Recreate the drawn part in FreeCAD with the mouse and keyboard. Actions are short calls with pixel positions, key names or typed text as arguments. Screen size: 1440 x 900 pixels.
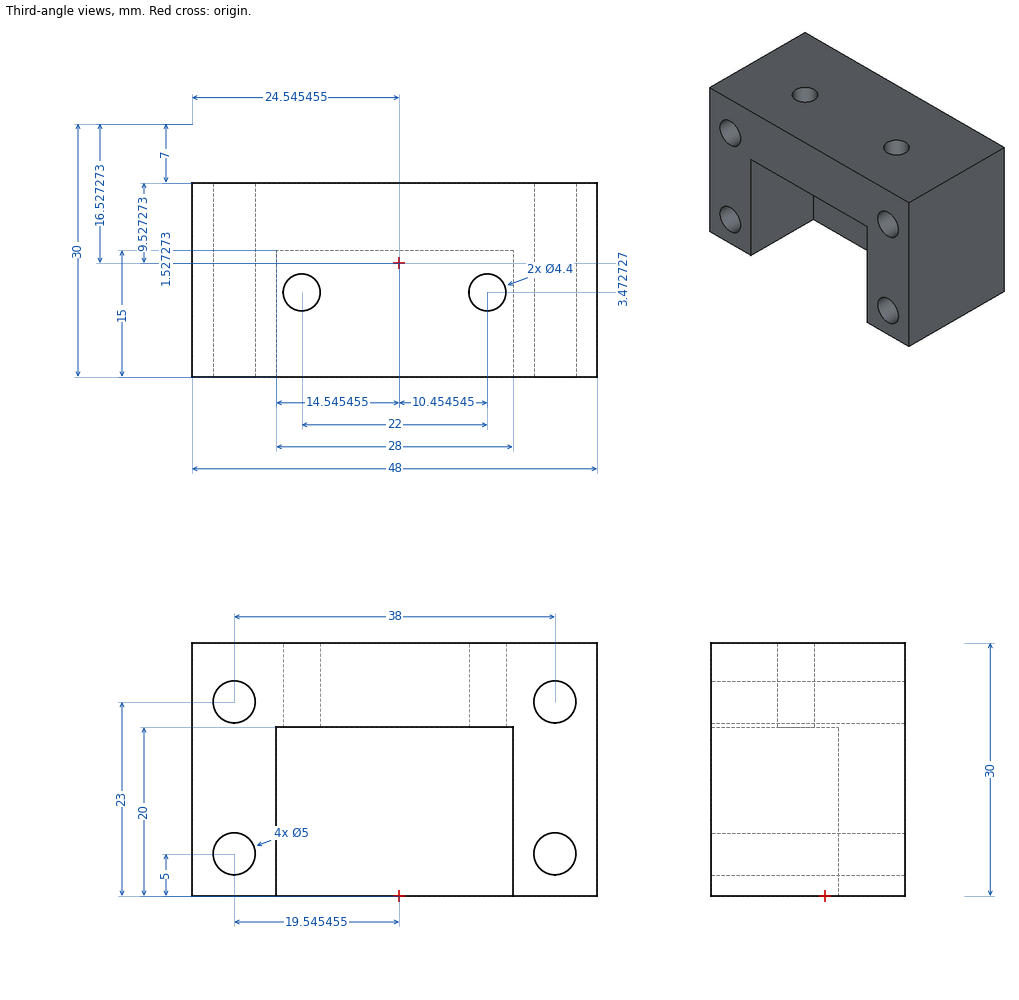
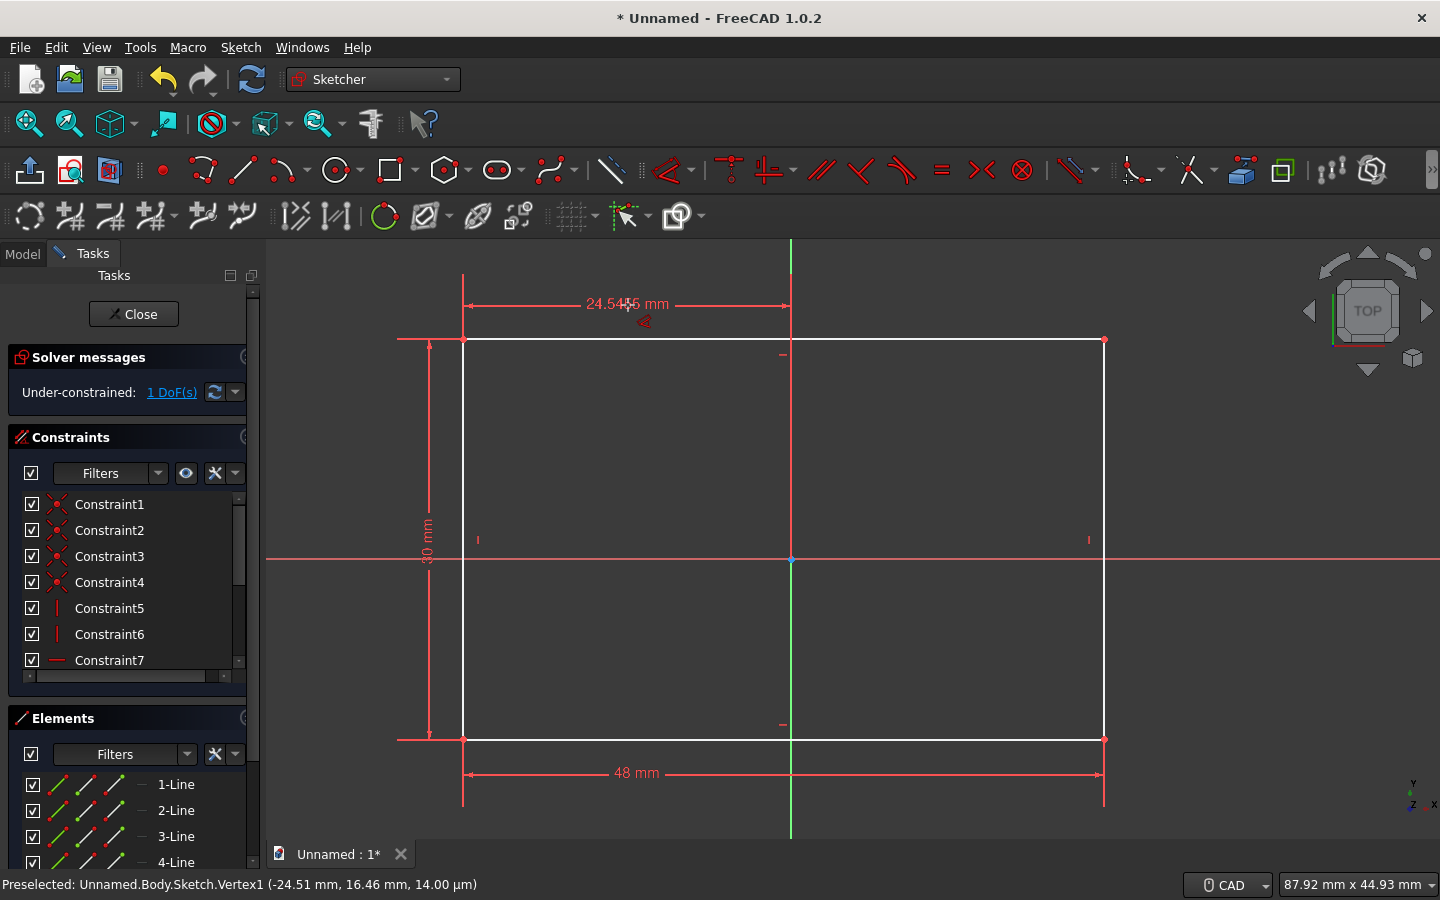
click(464, 339)
click(430, 449)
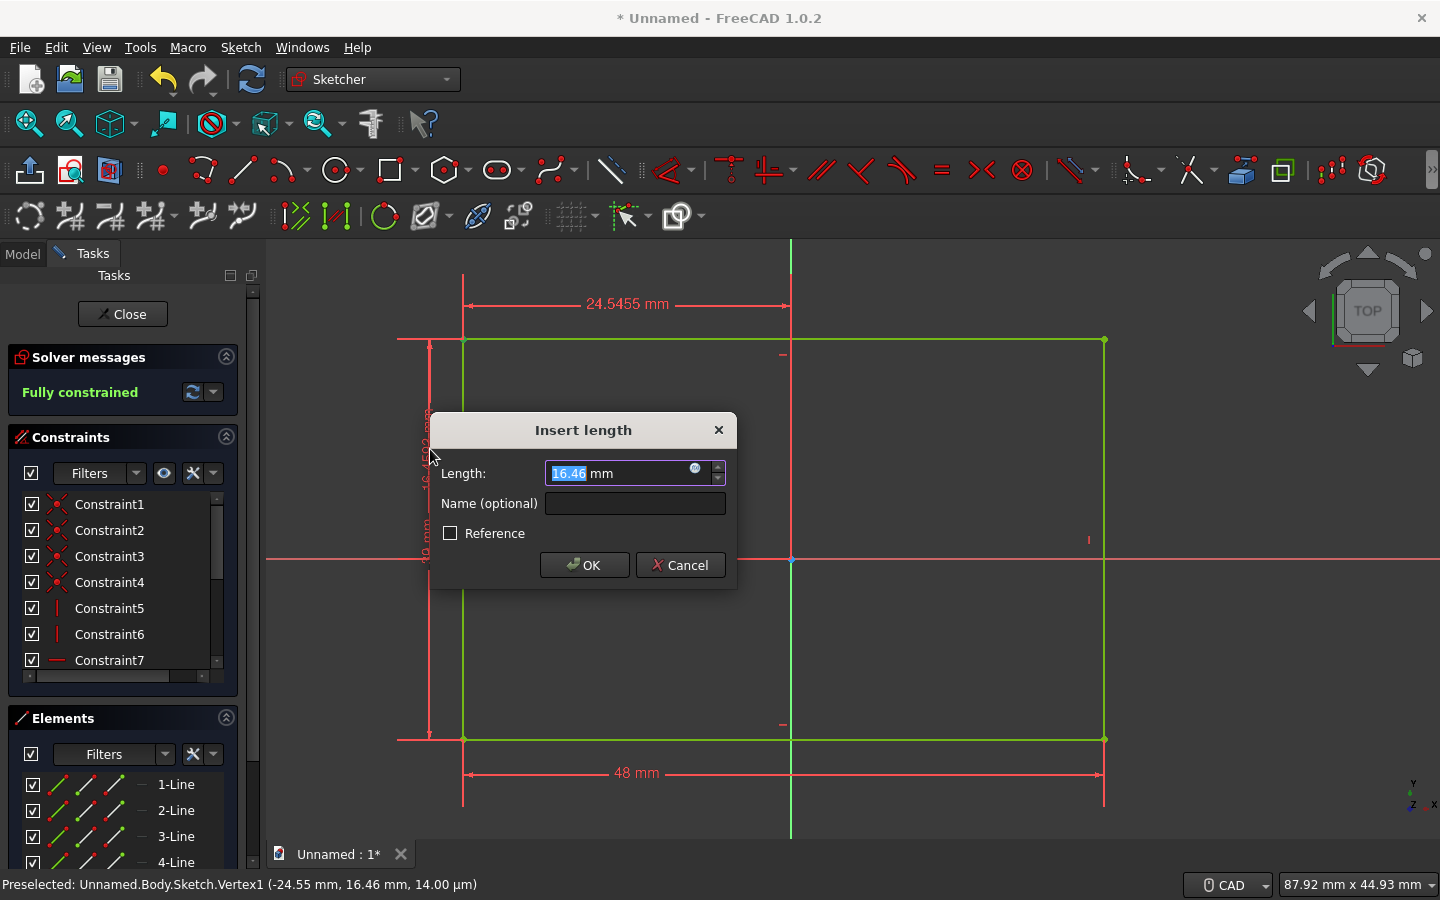
text(16.527273)
key(Return)
key(Escape)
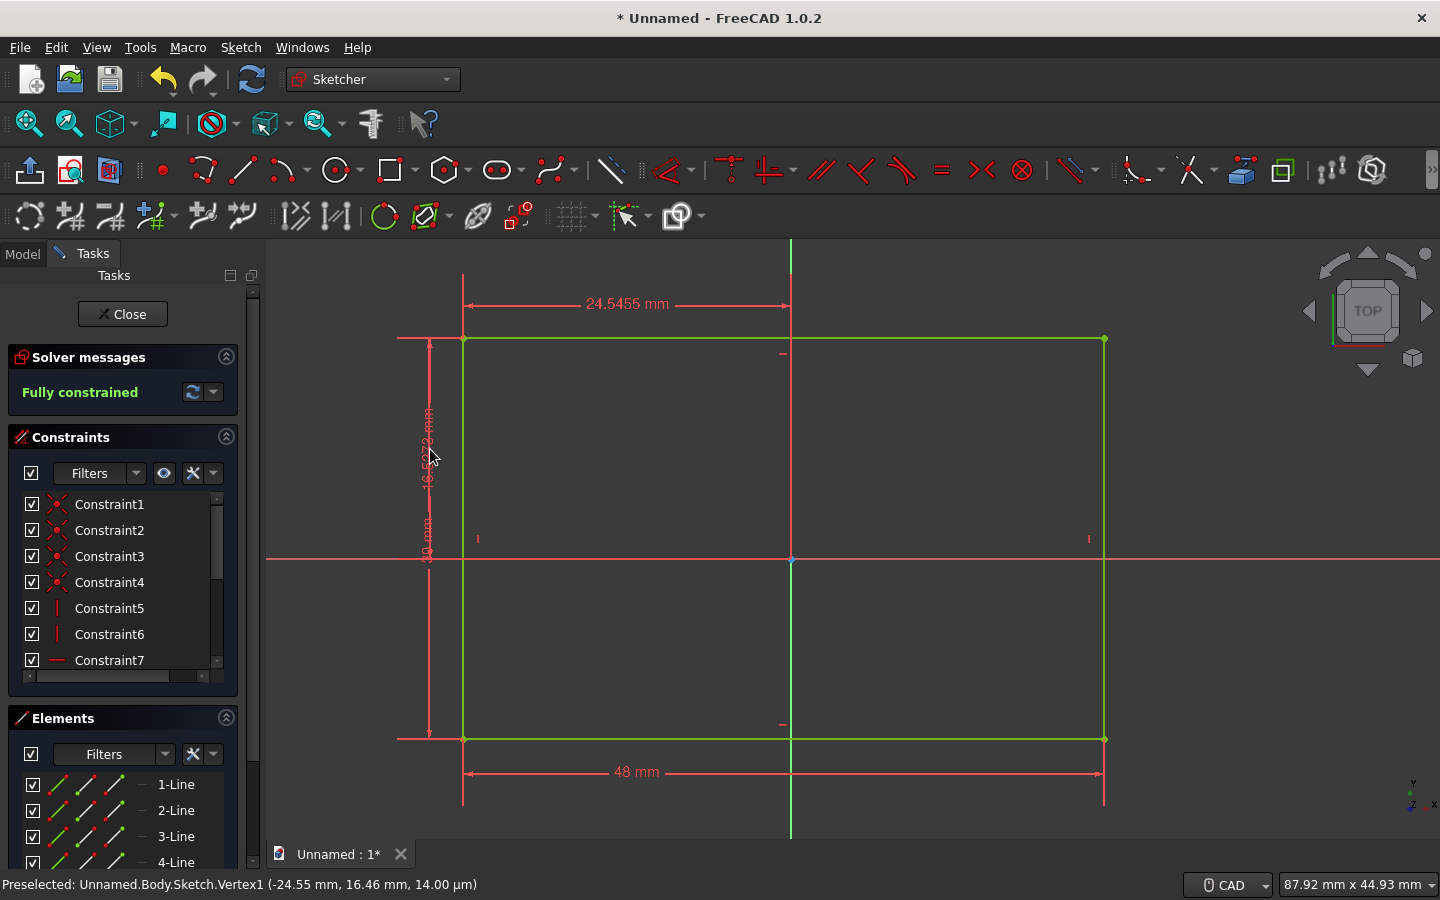
click(123, 314)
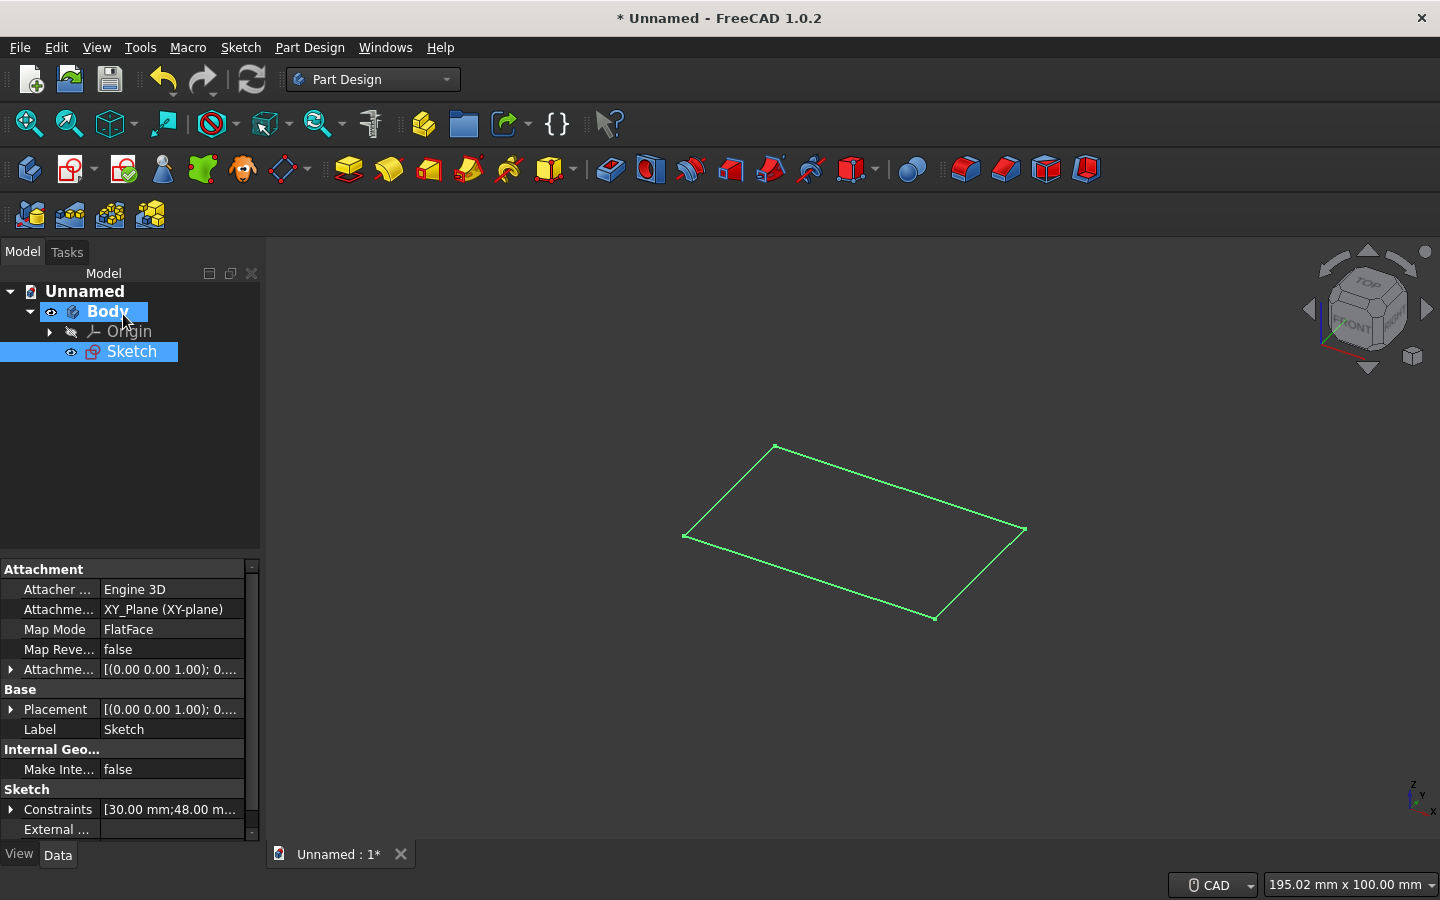
click(350, 170)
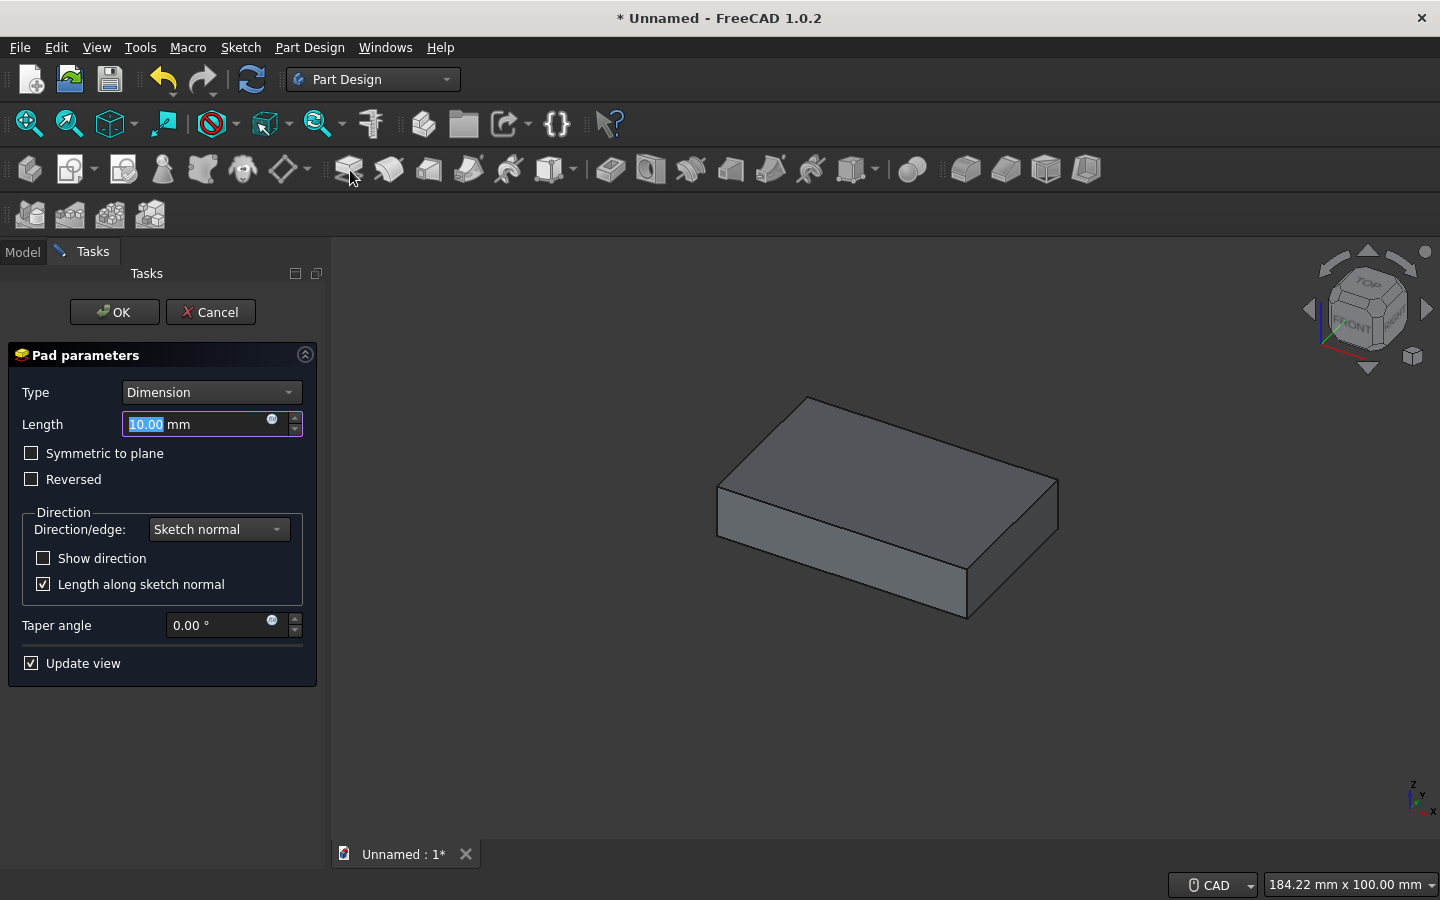
text(30)
key(Tab)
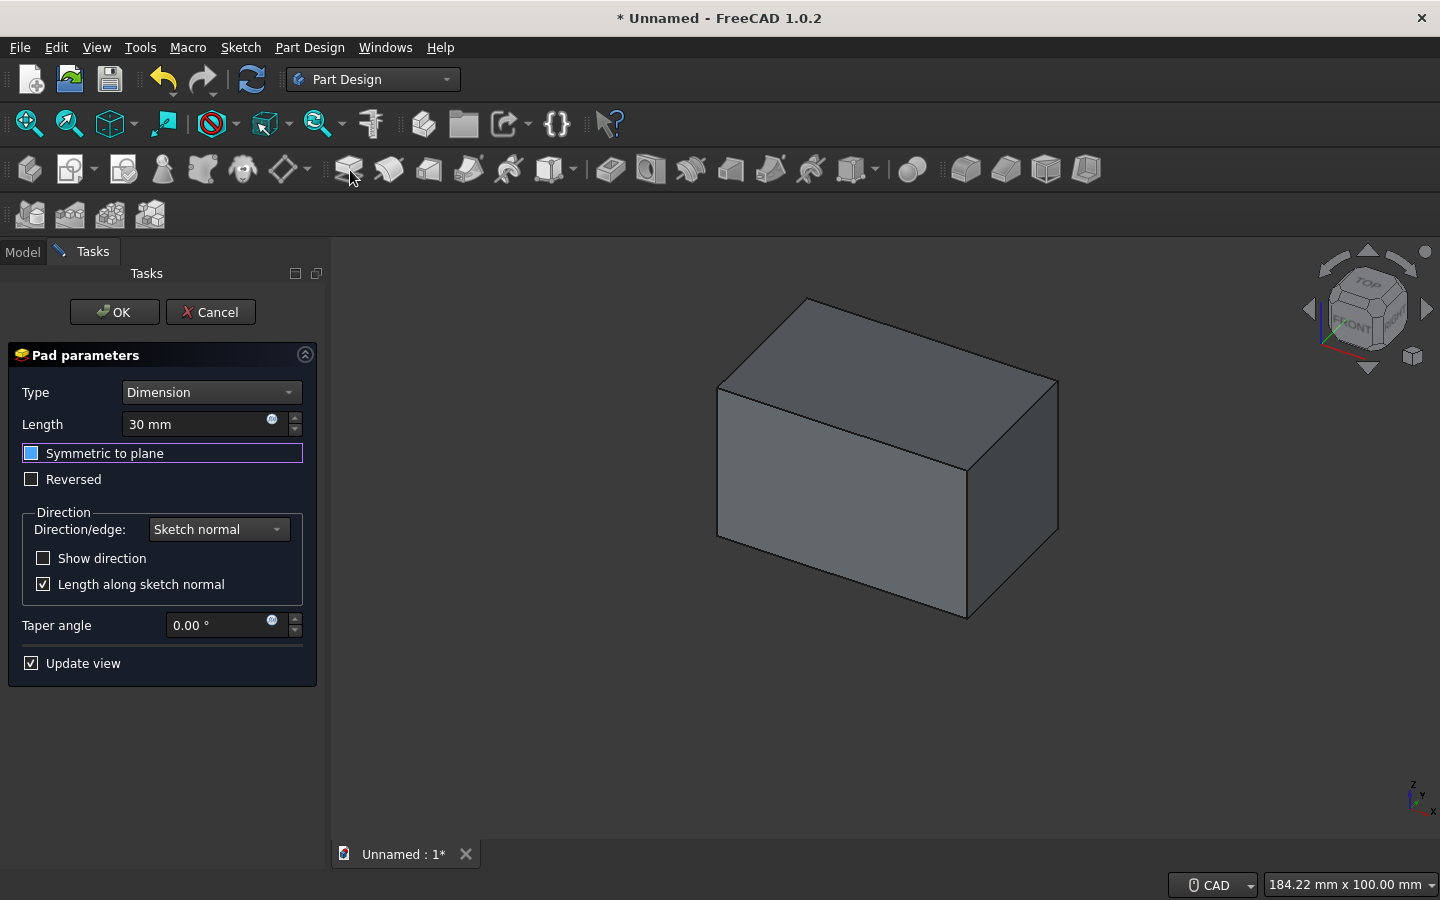
click(115, 312)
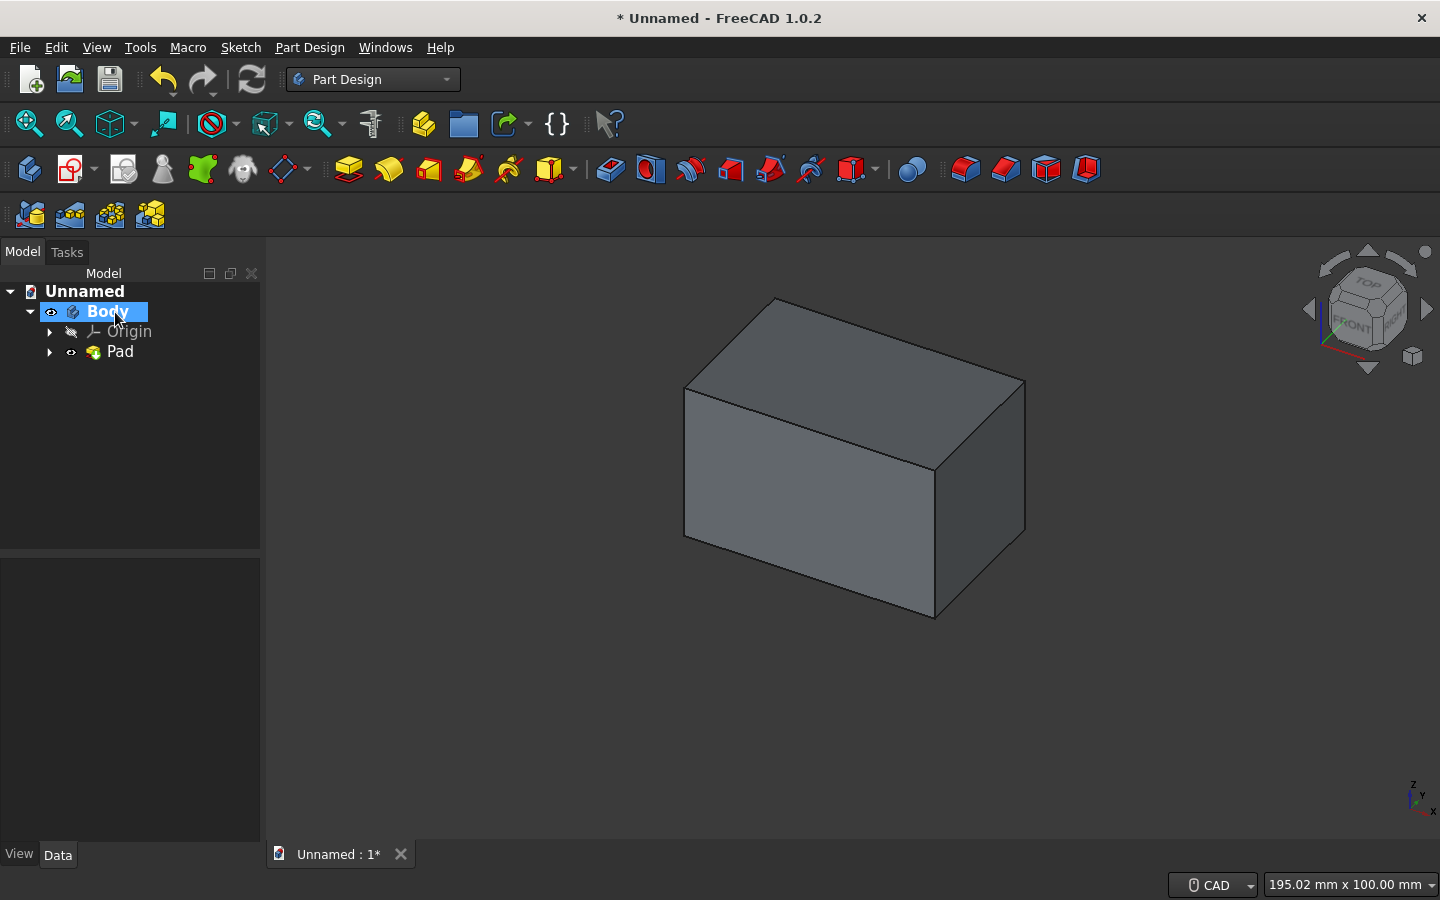
click(70, 170)